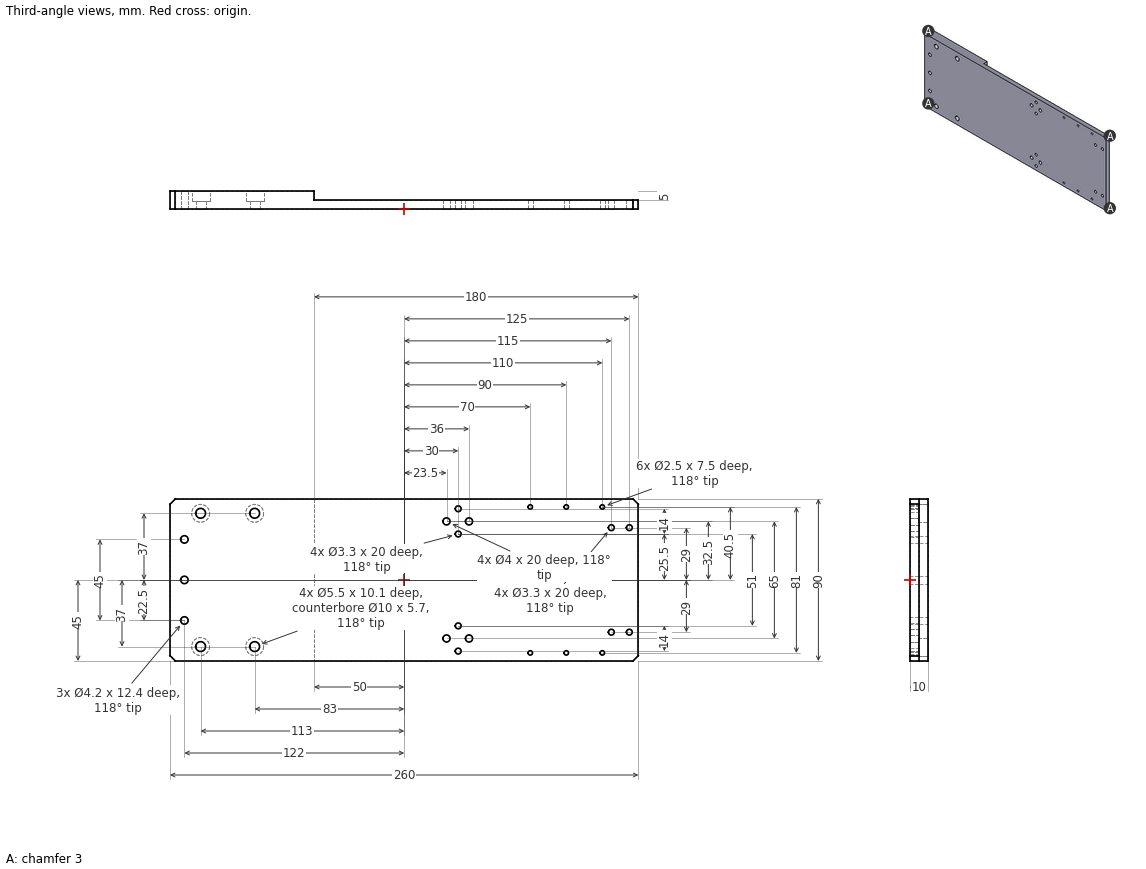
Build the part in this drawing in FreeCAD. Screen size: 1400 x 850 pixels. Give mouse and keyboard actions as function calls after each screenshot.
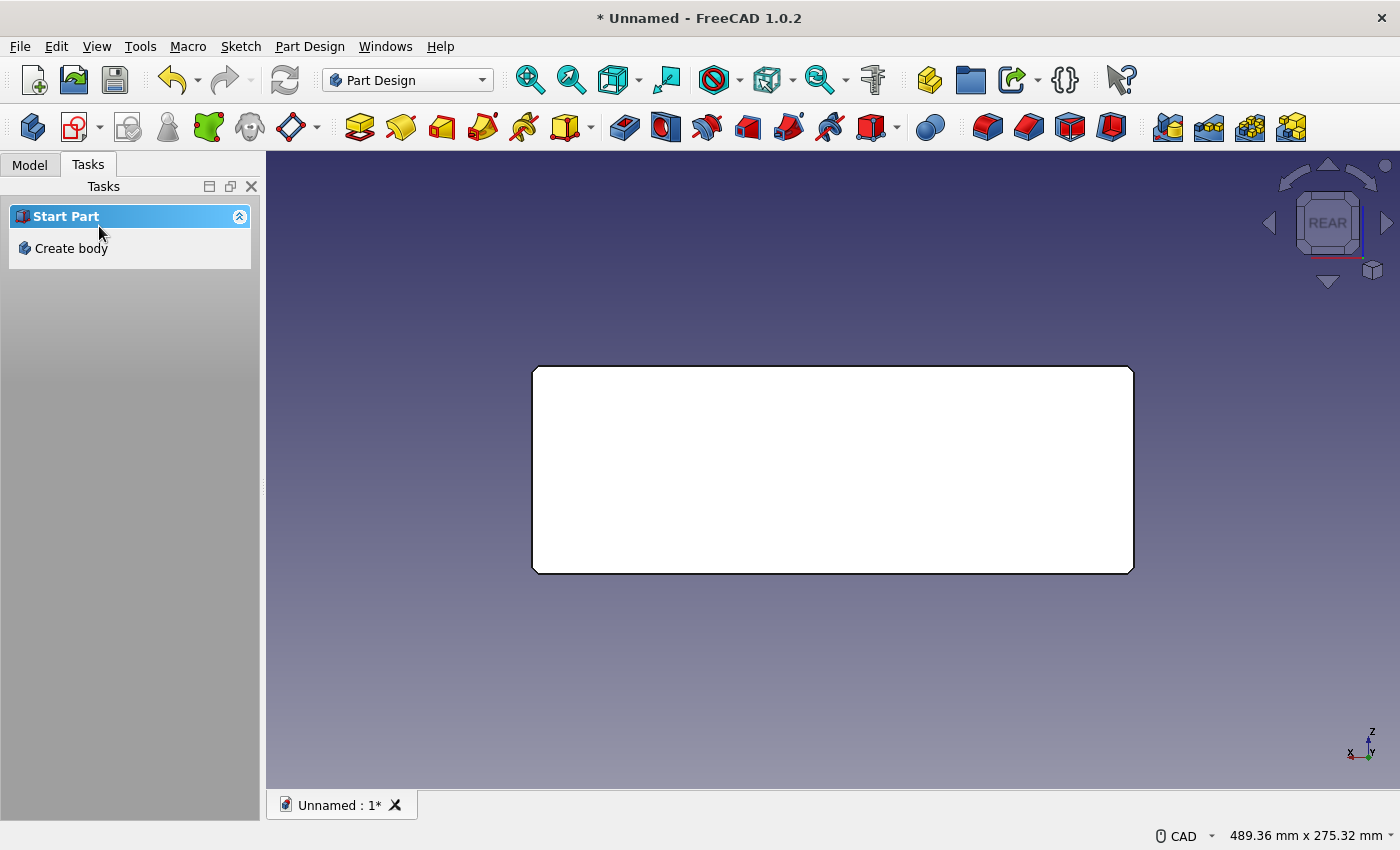
click(661, 469)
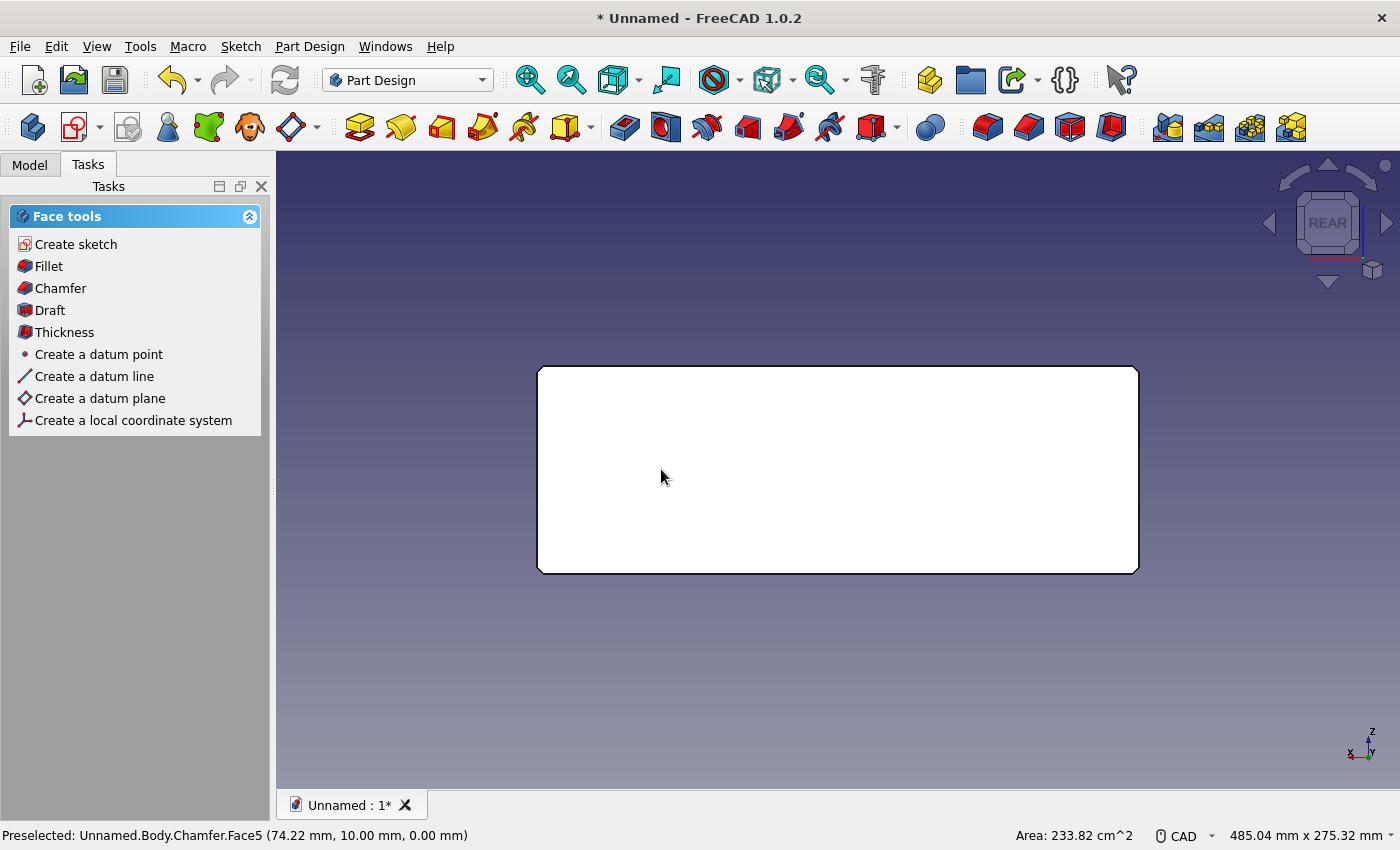
click(74, 128)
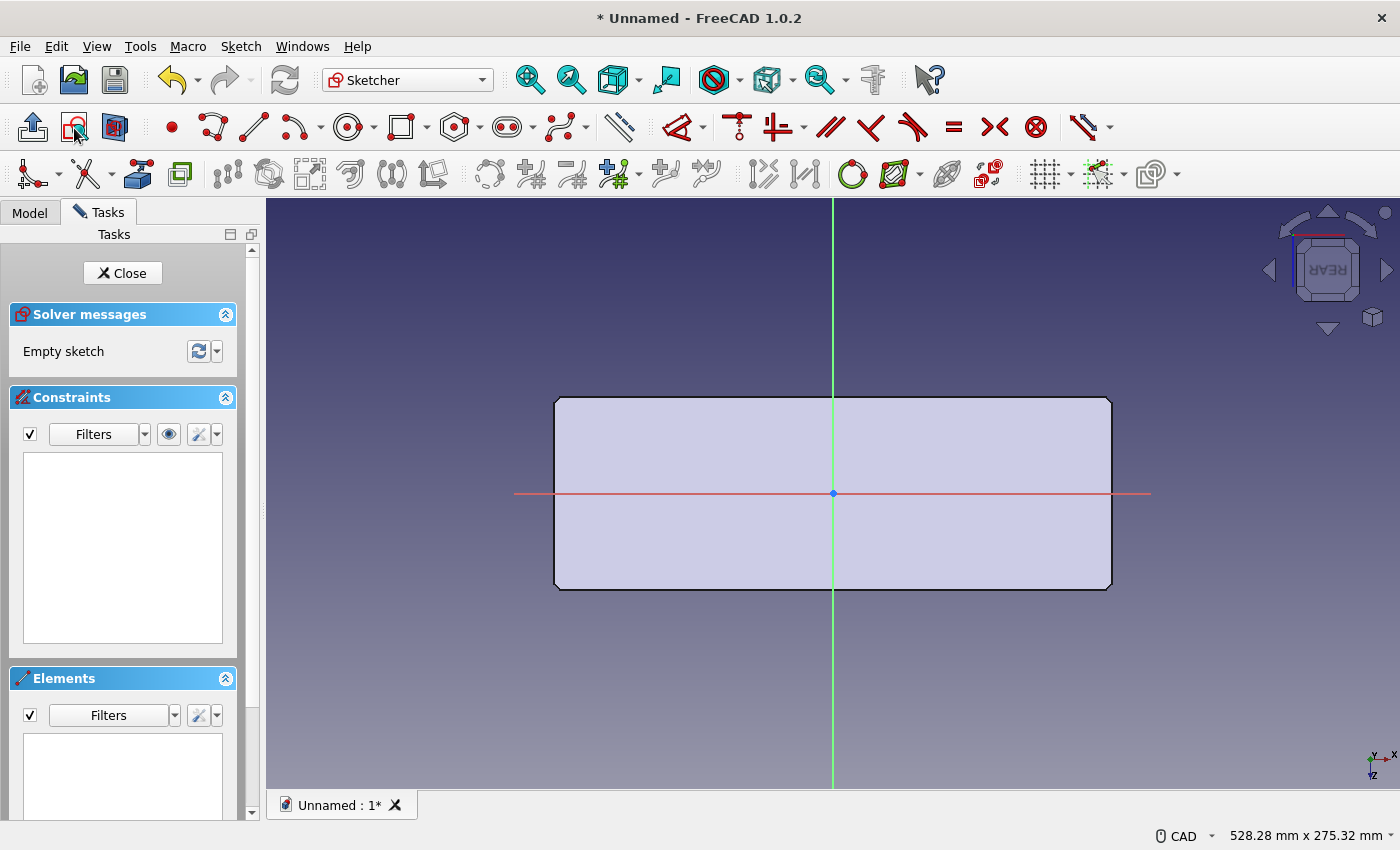
scroll(663, 494, up, 4)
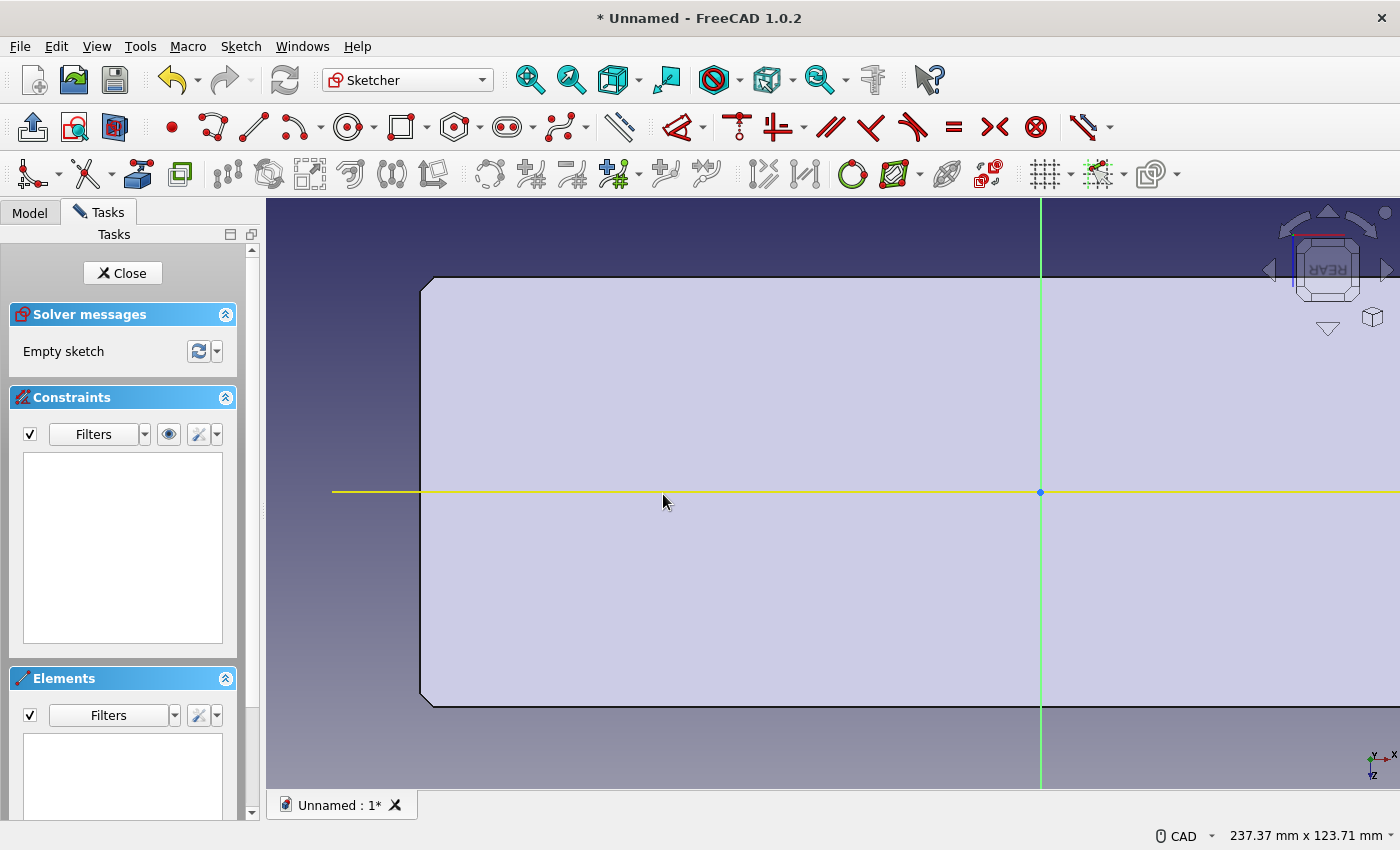
click(348, 128)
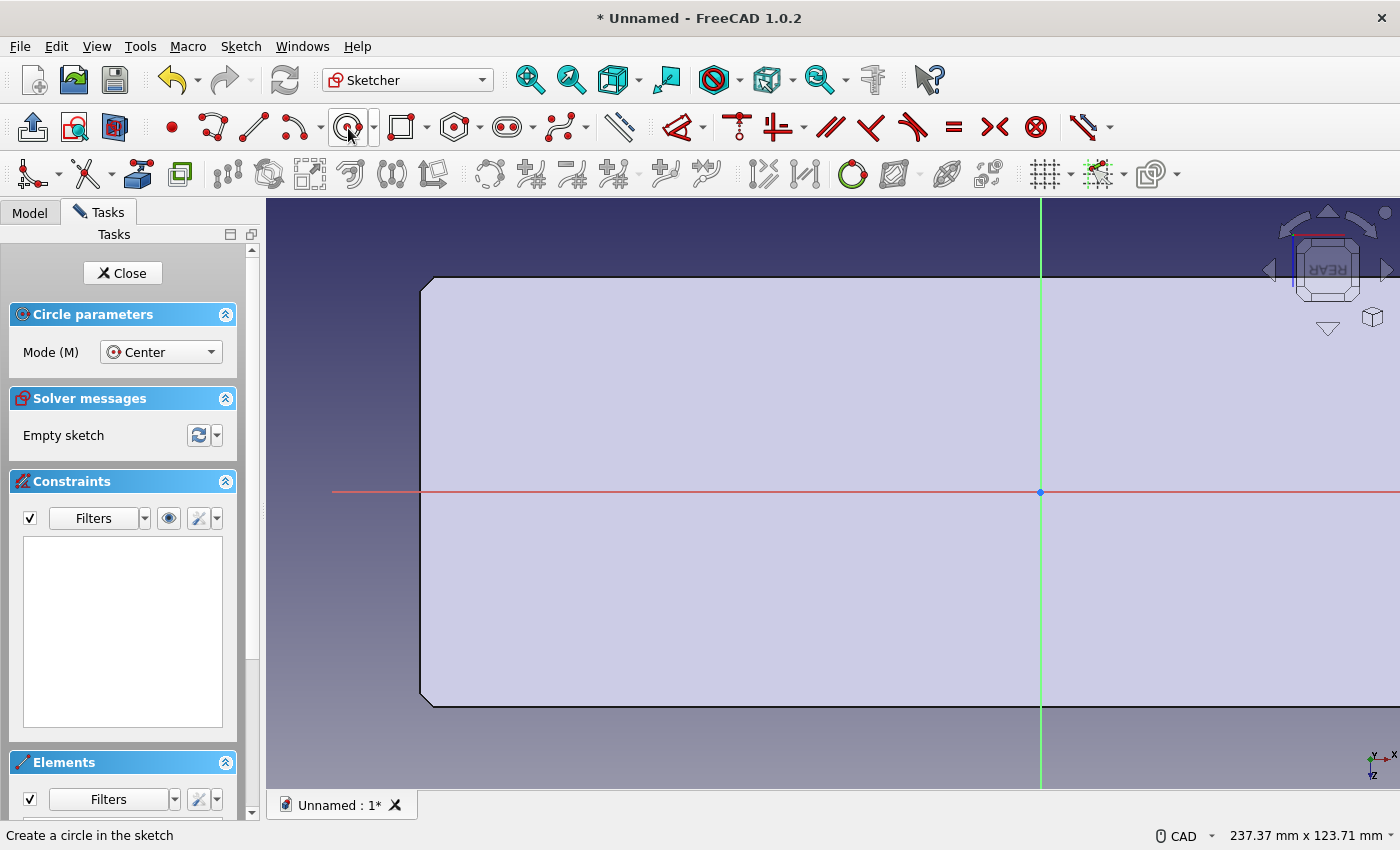
scroll(644, 316, up, 3)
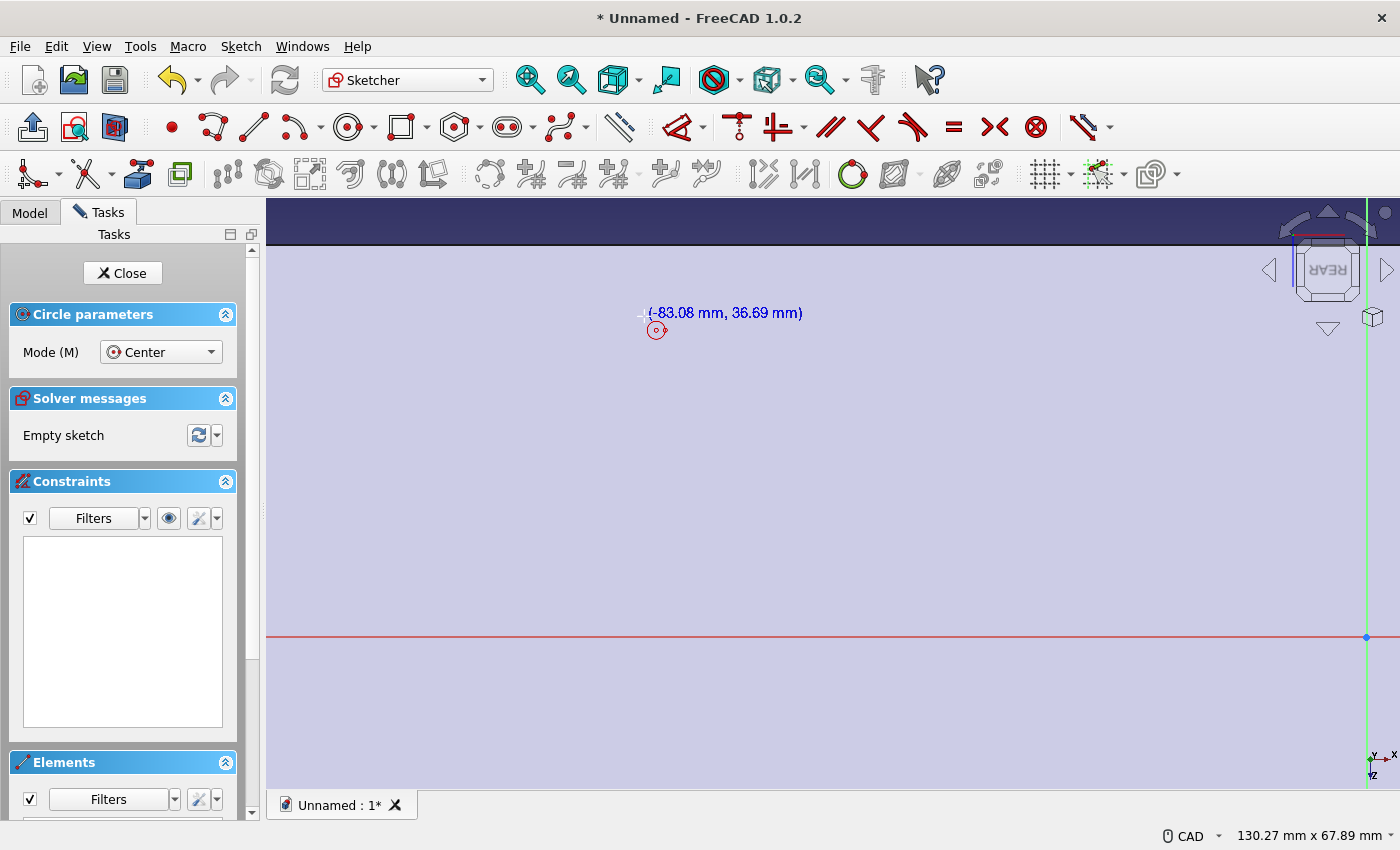
click(644, 315)
click(661, 298)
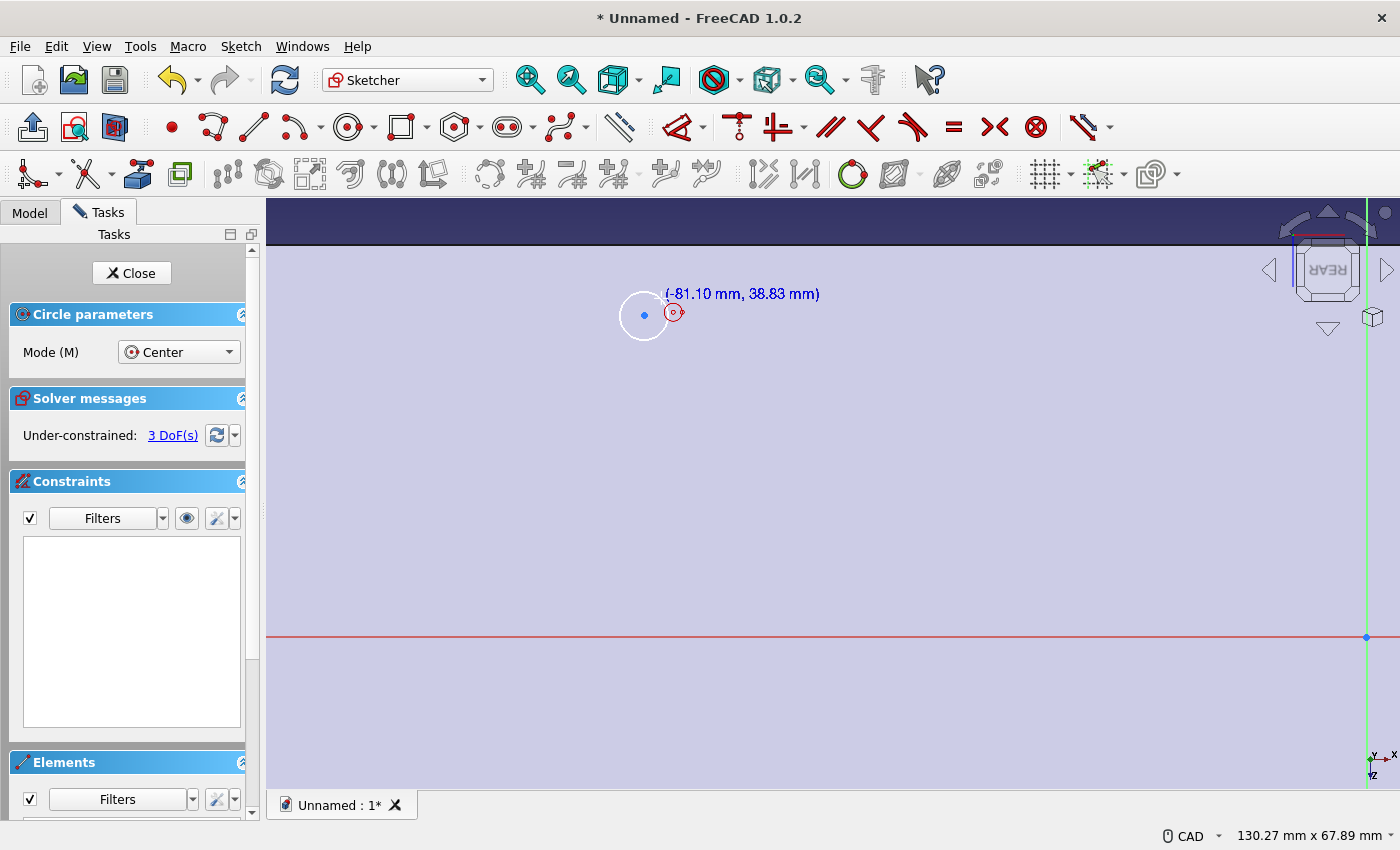
click(383, 315)
click(400, 298)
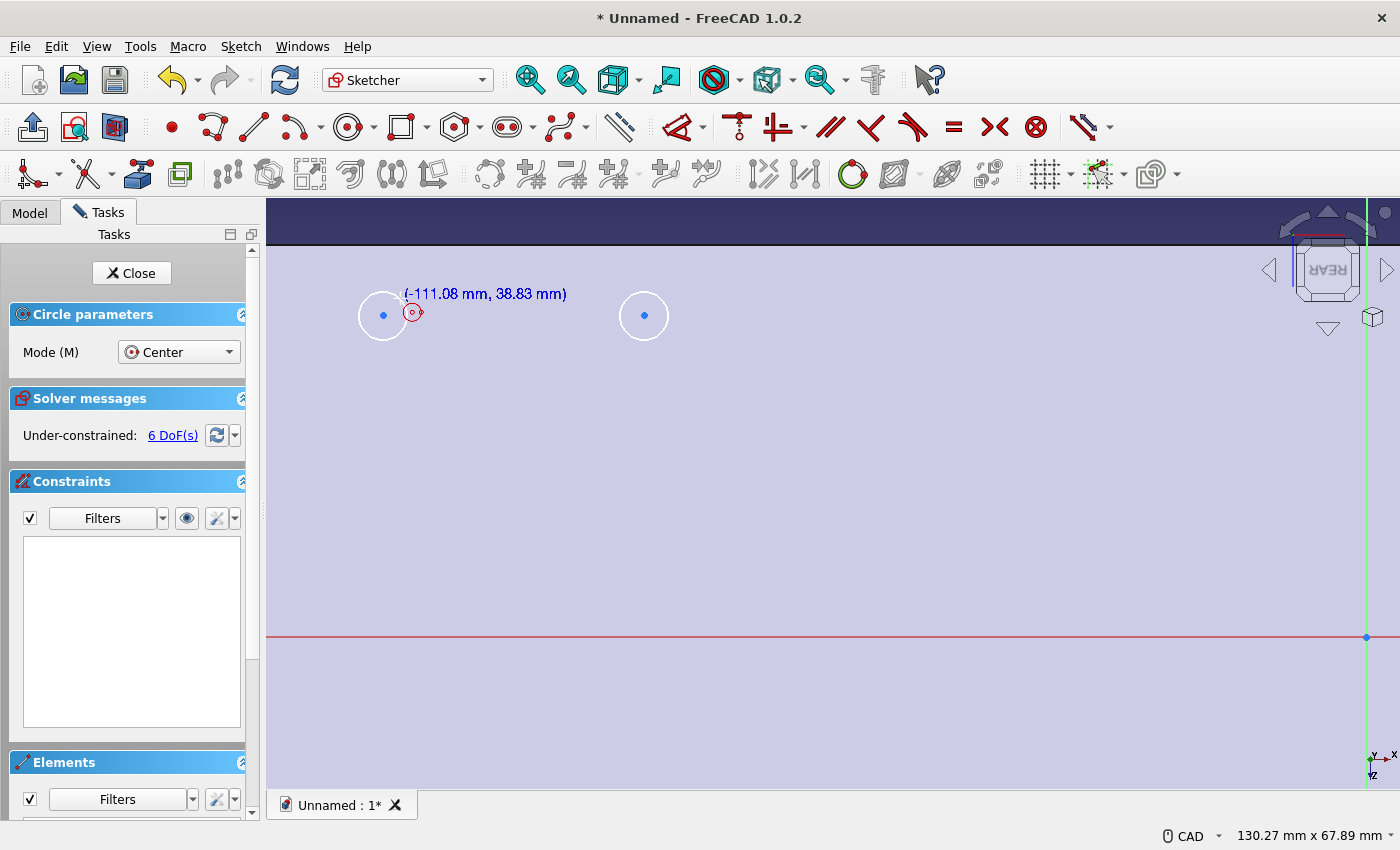
scroll(645, 319, down, 3)